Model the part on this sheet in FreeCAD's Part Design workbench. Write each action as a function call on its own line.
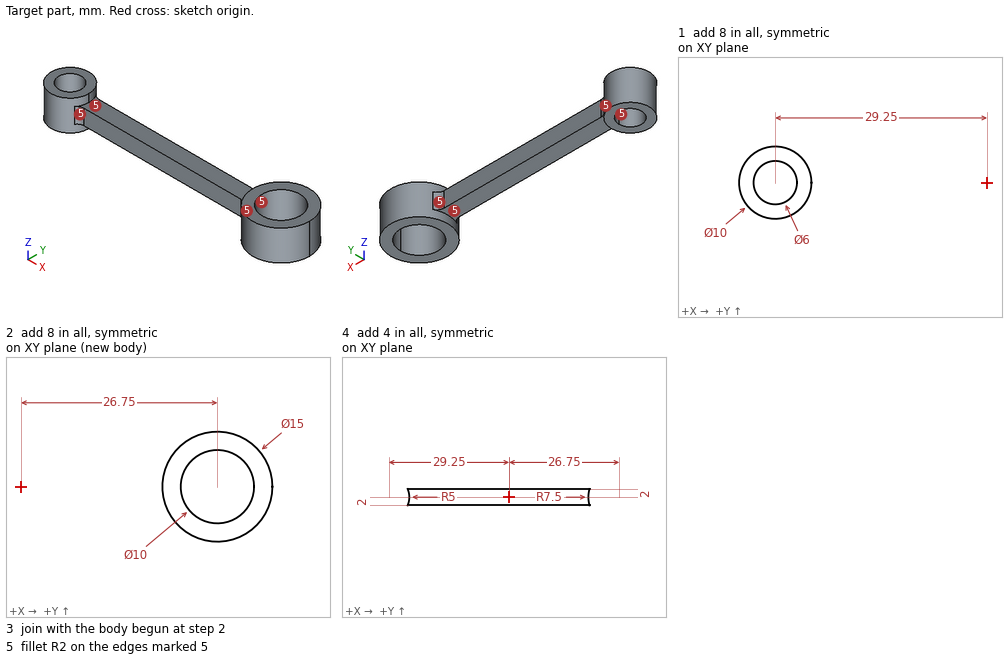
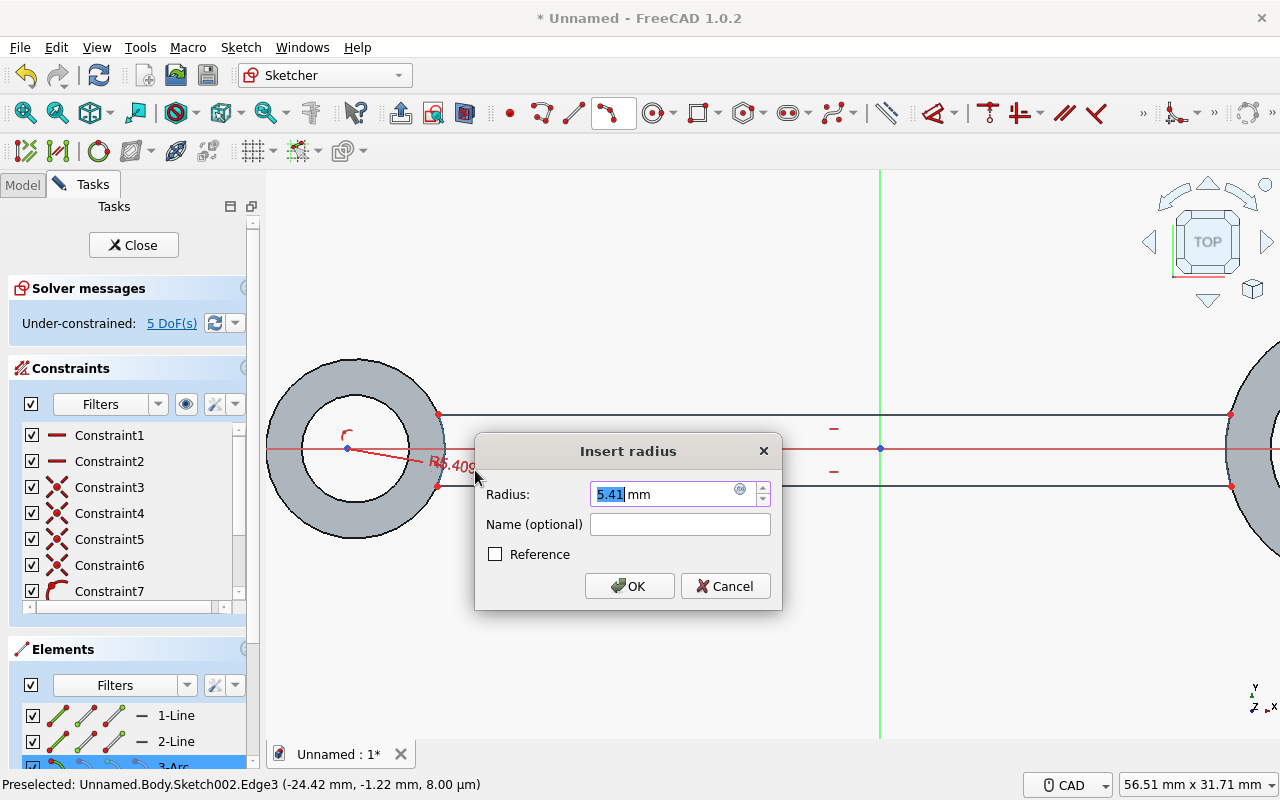
text(5)
key(Return)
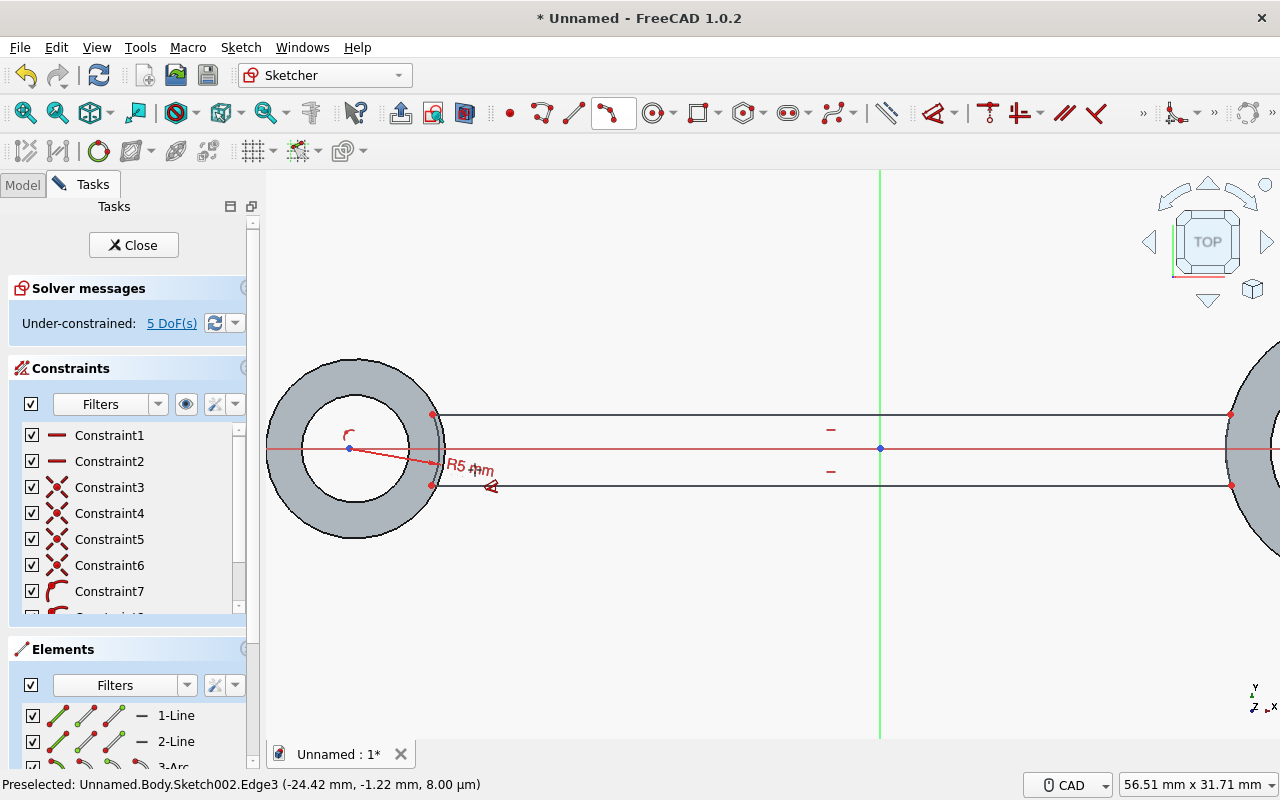
scroll(441, 466, down, 2)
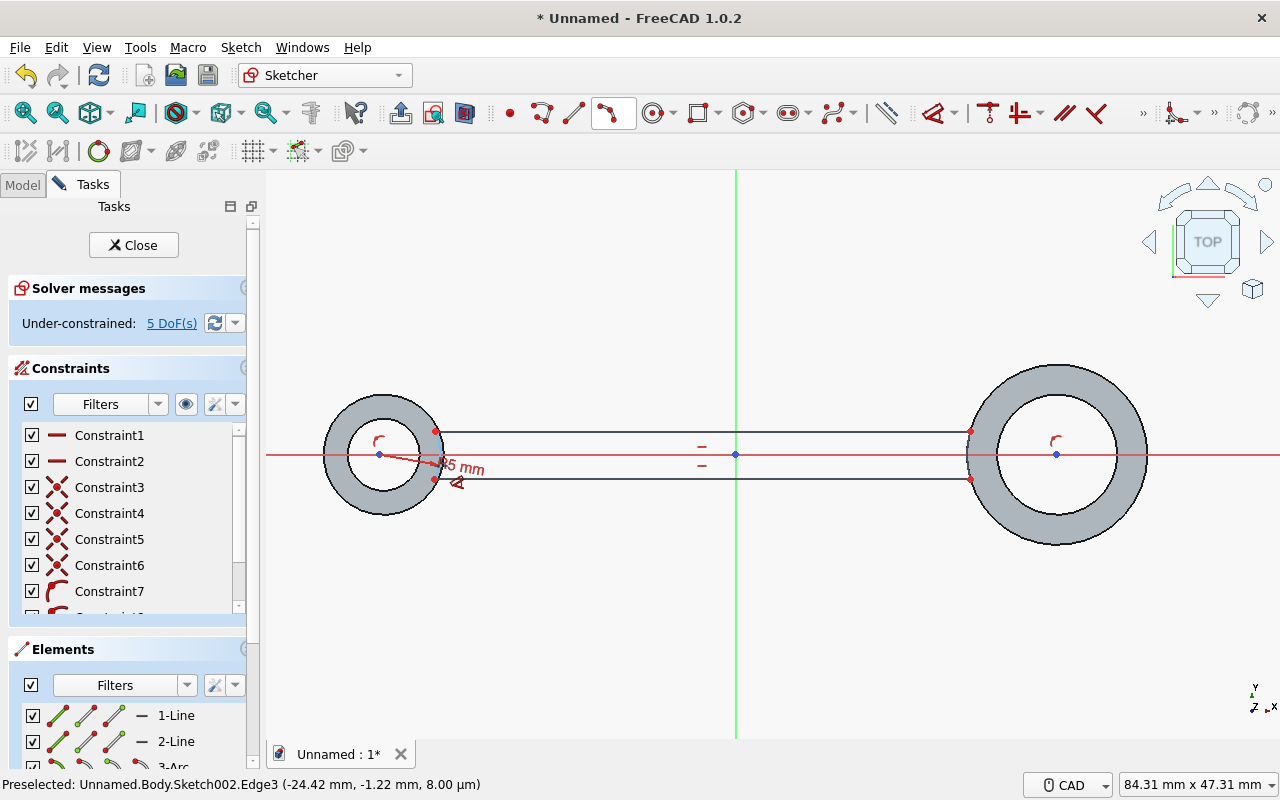
scroll(968, 446, up, 3)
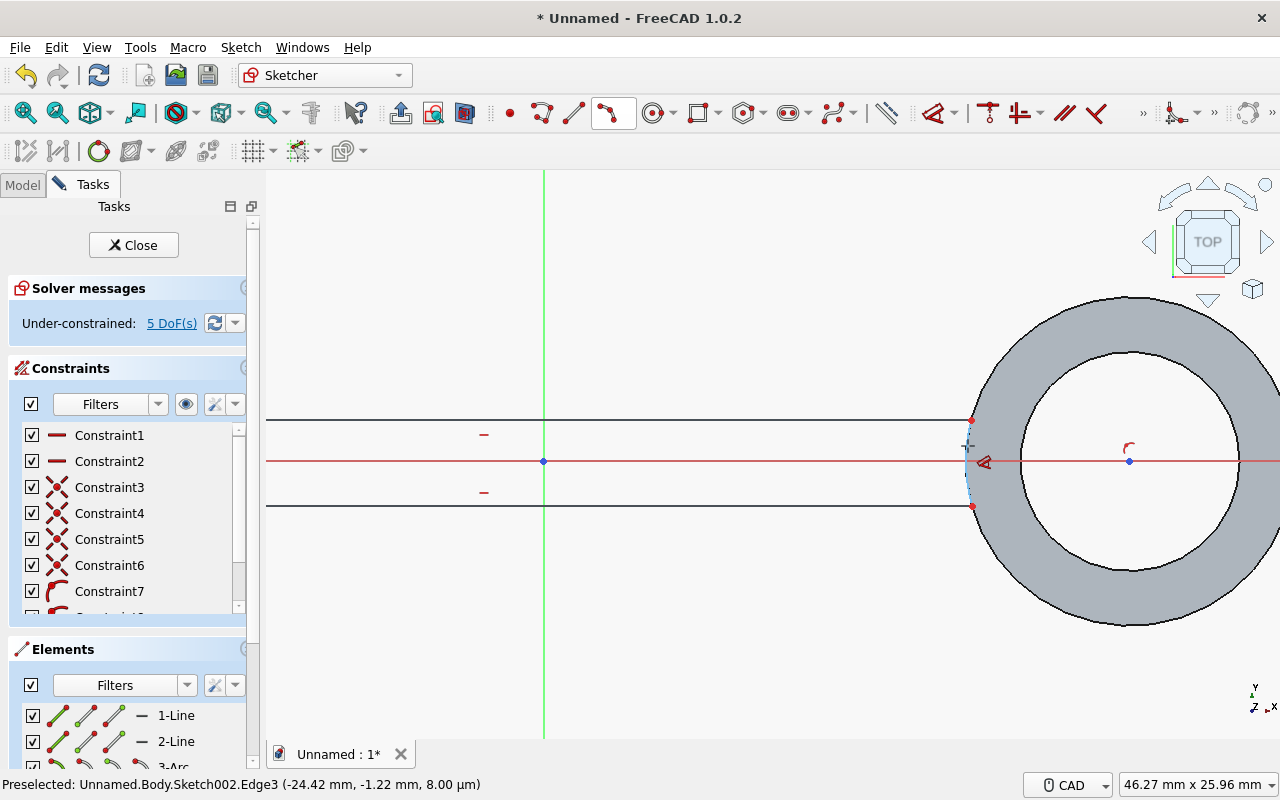
click(967, 446)
click(935, 443)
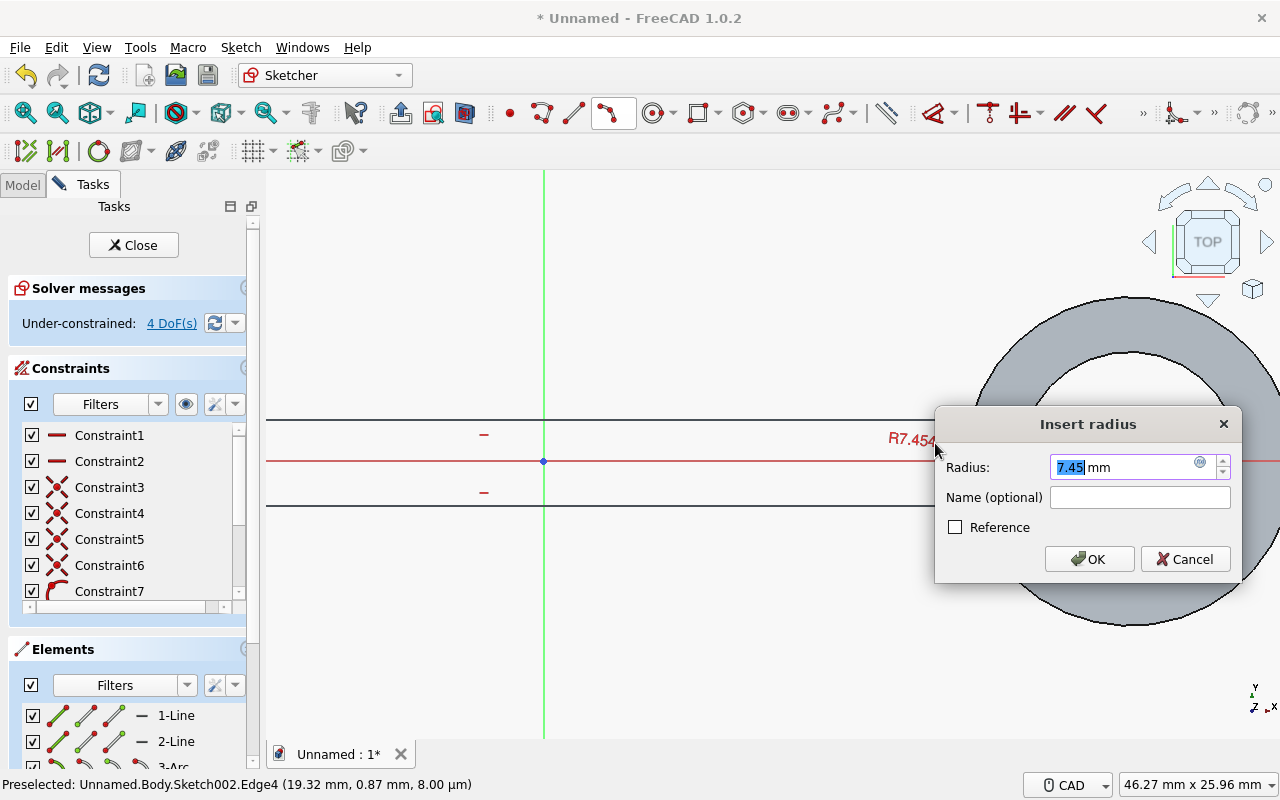
text(7.5)
key(Return)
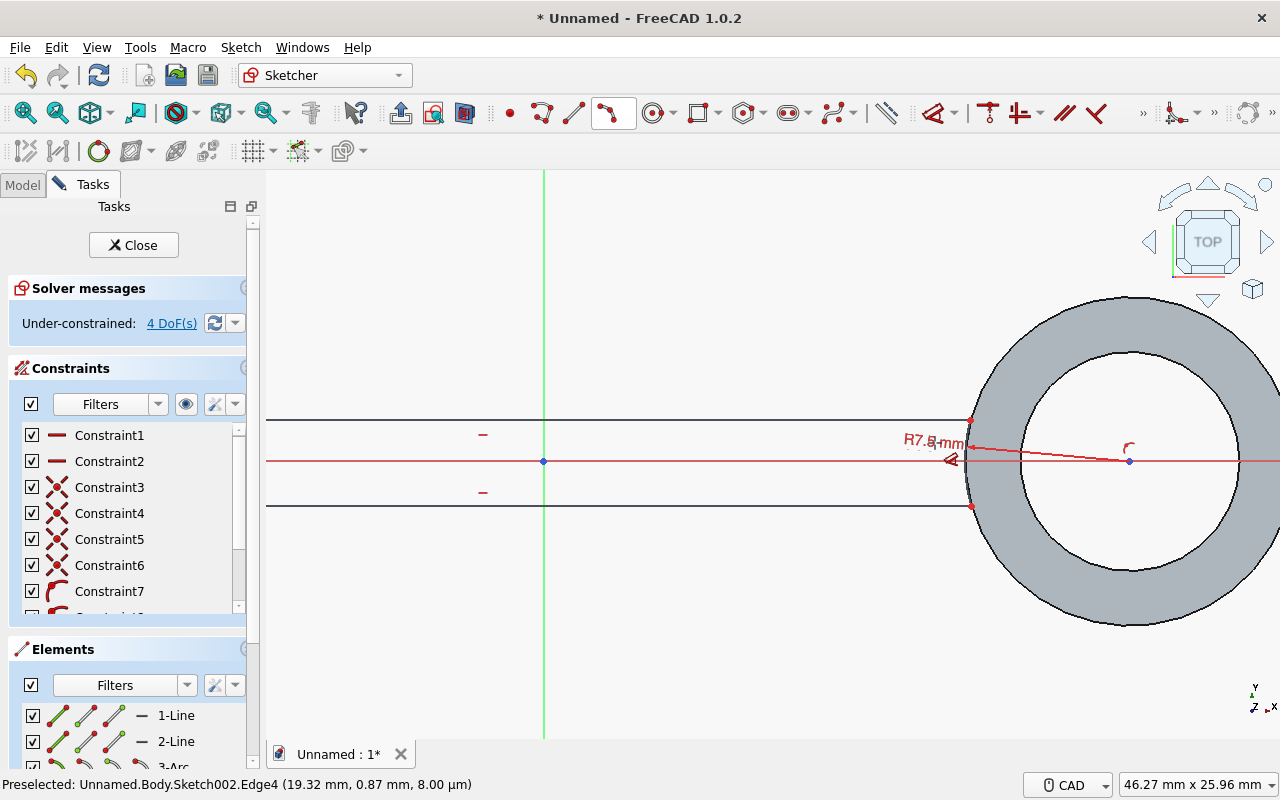
click(970, 420)
click(510, 441)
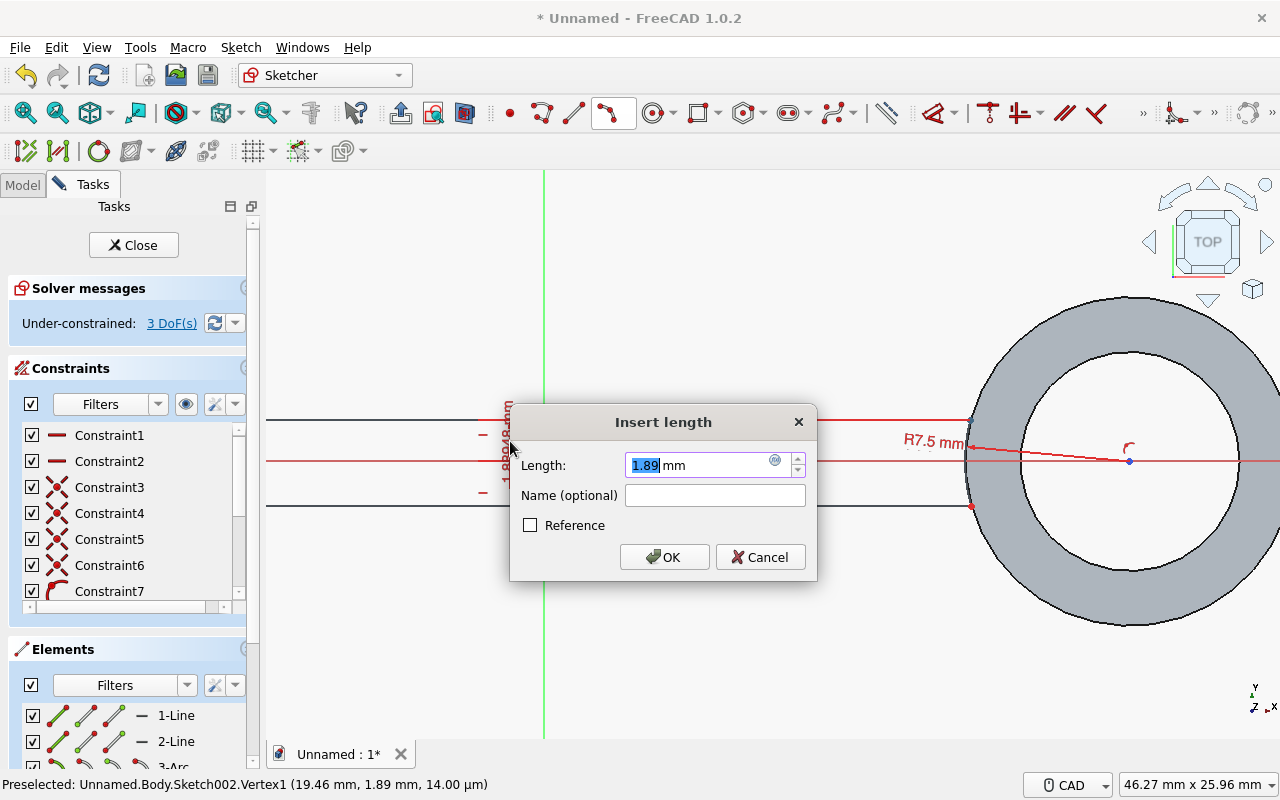
text(2)
key(Return)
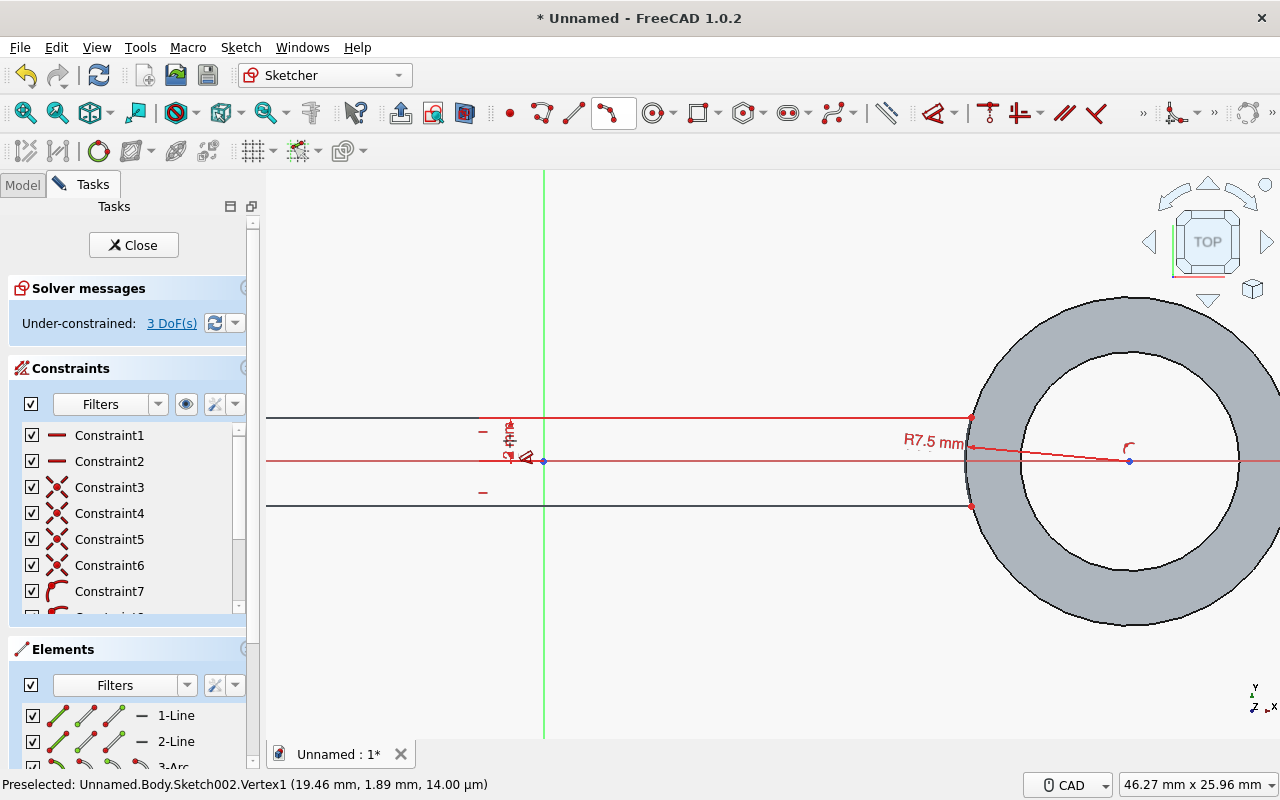
scroll(969, 446, down, 3)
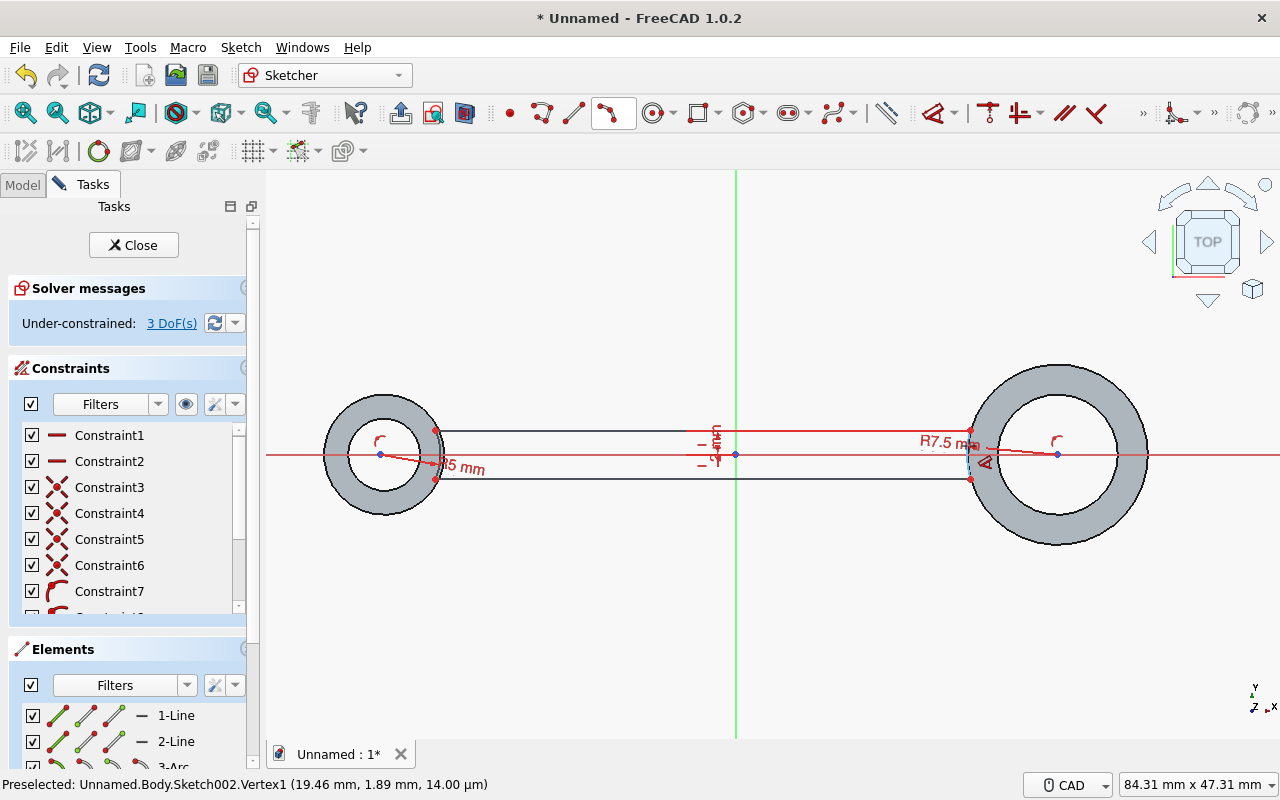
scroll(435, 479, up, 3)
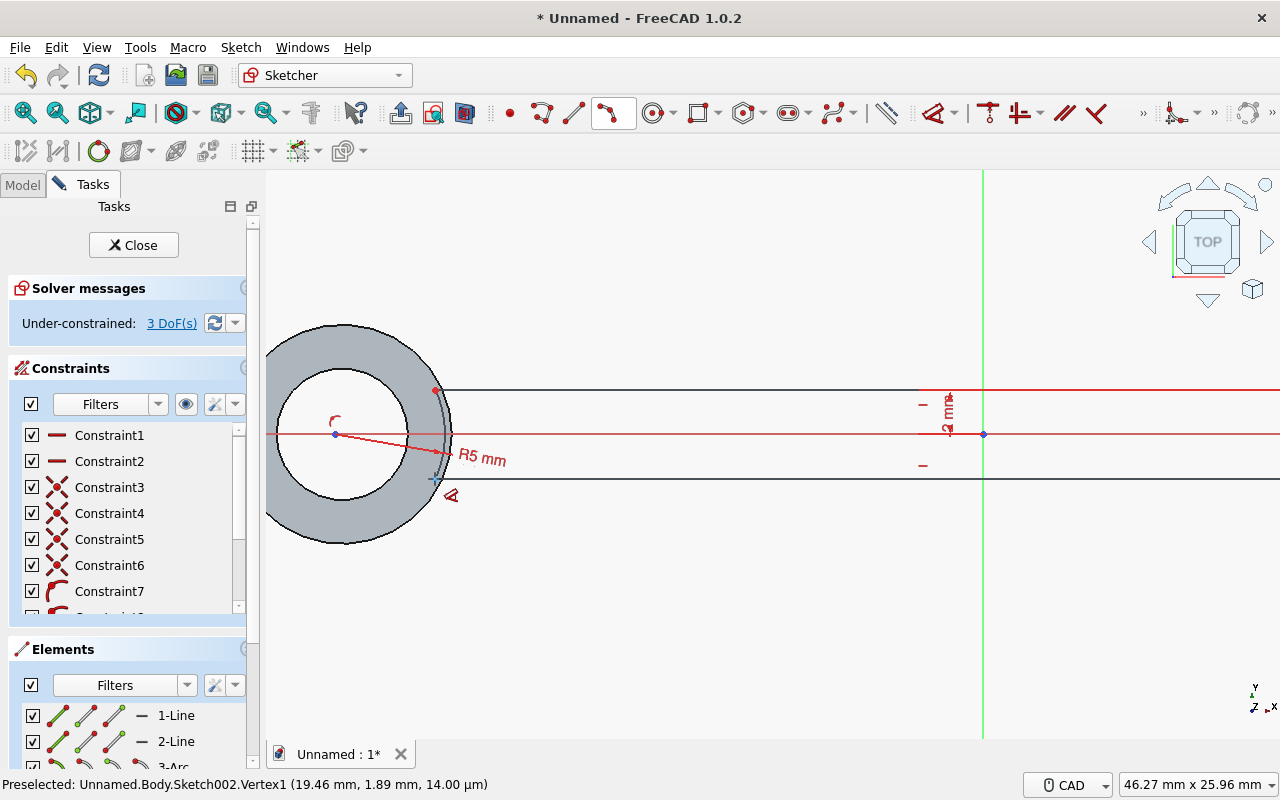
click(435, 479)
click(401, 457)